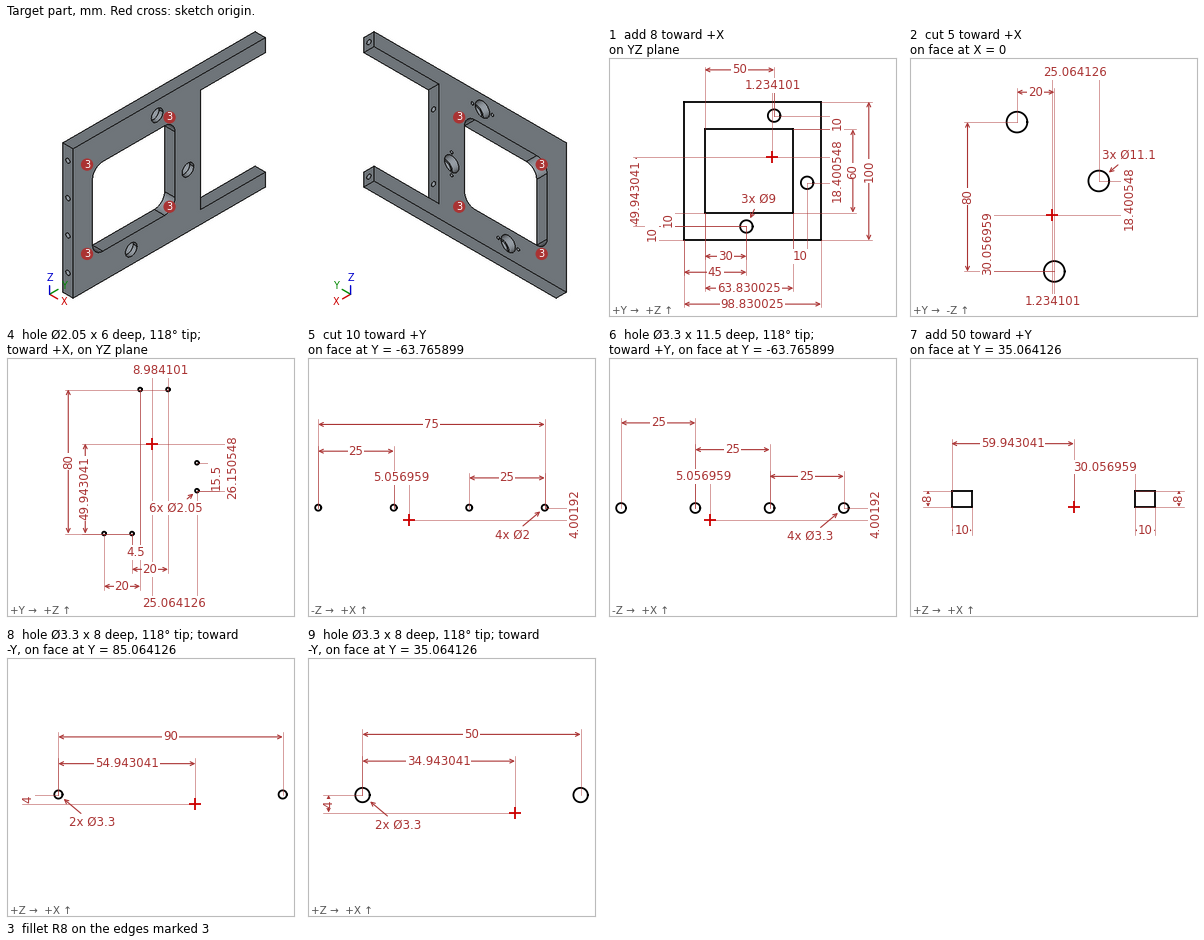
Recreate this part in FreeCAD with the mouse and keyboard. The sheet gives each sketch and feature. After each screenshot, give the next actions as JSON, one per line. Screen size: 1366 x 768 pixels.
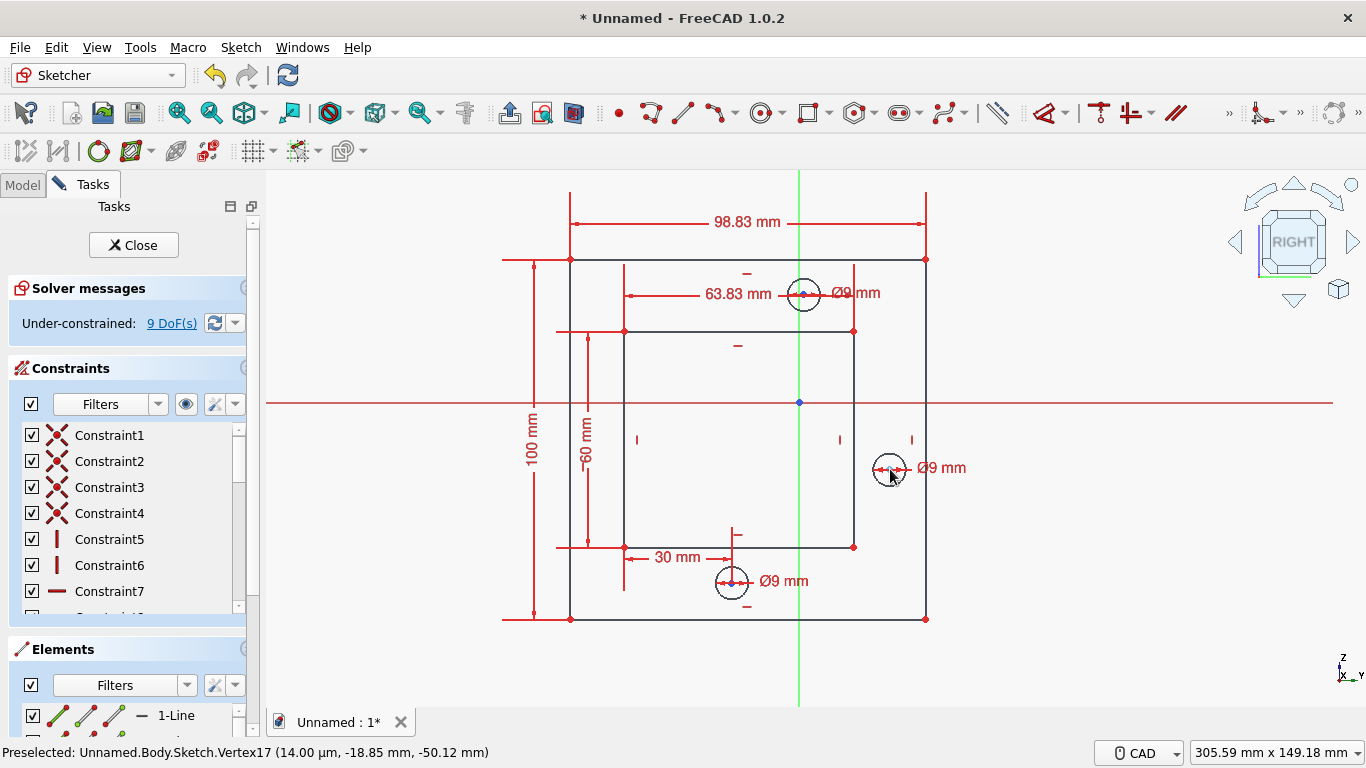
{"action": "left_click", "coordinate": [570, 620]}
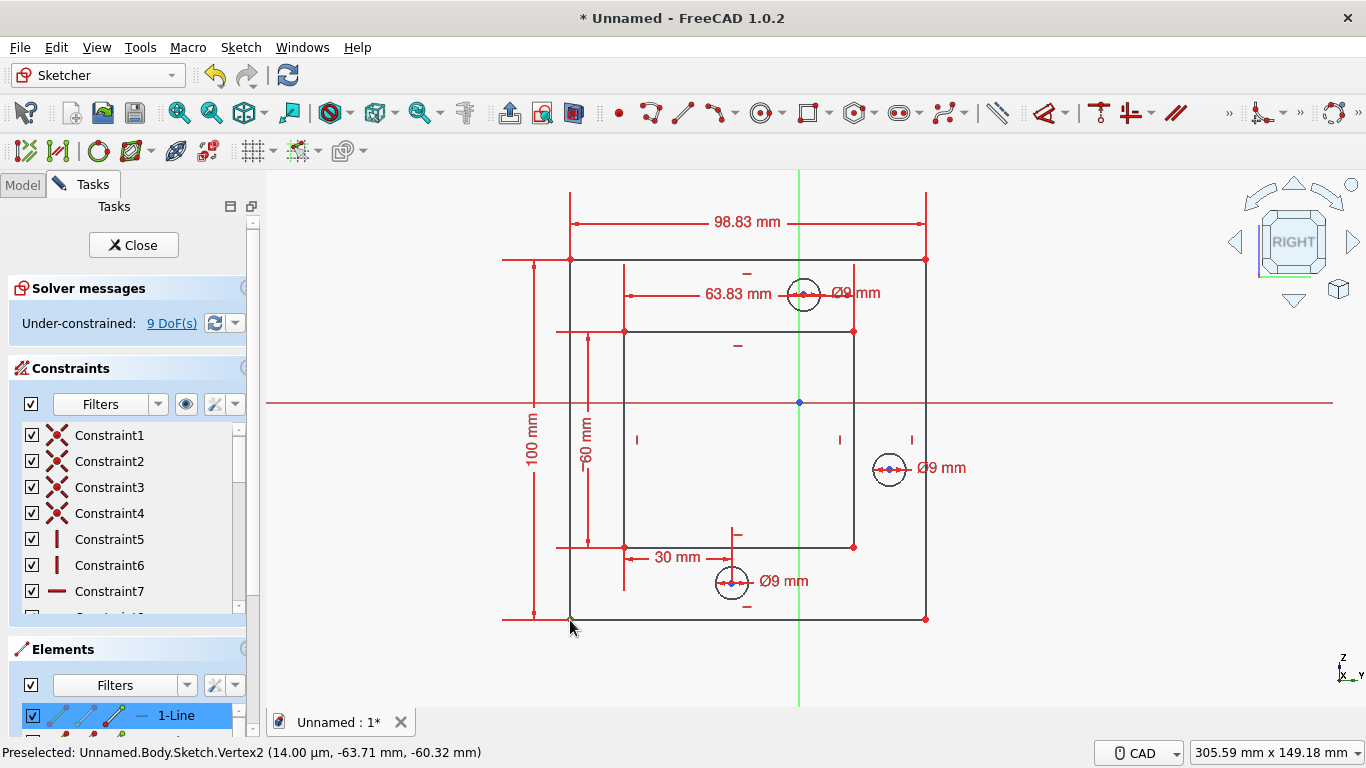
{"action": "left_click", "coordinate": [732, 583]}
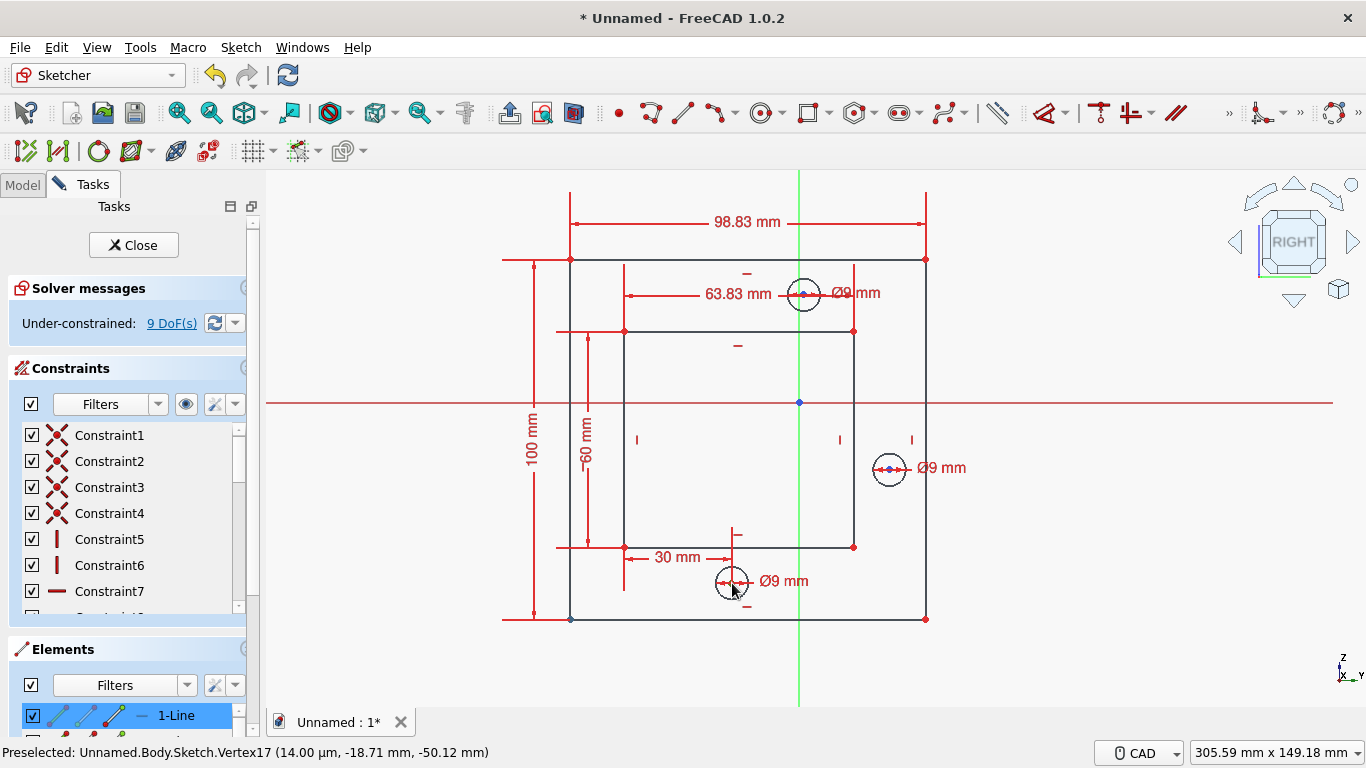
{"action": "key", "text": "l"}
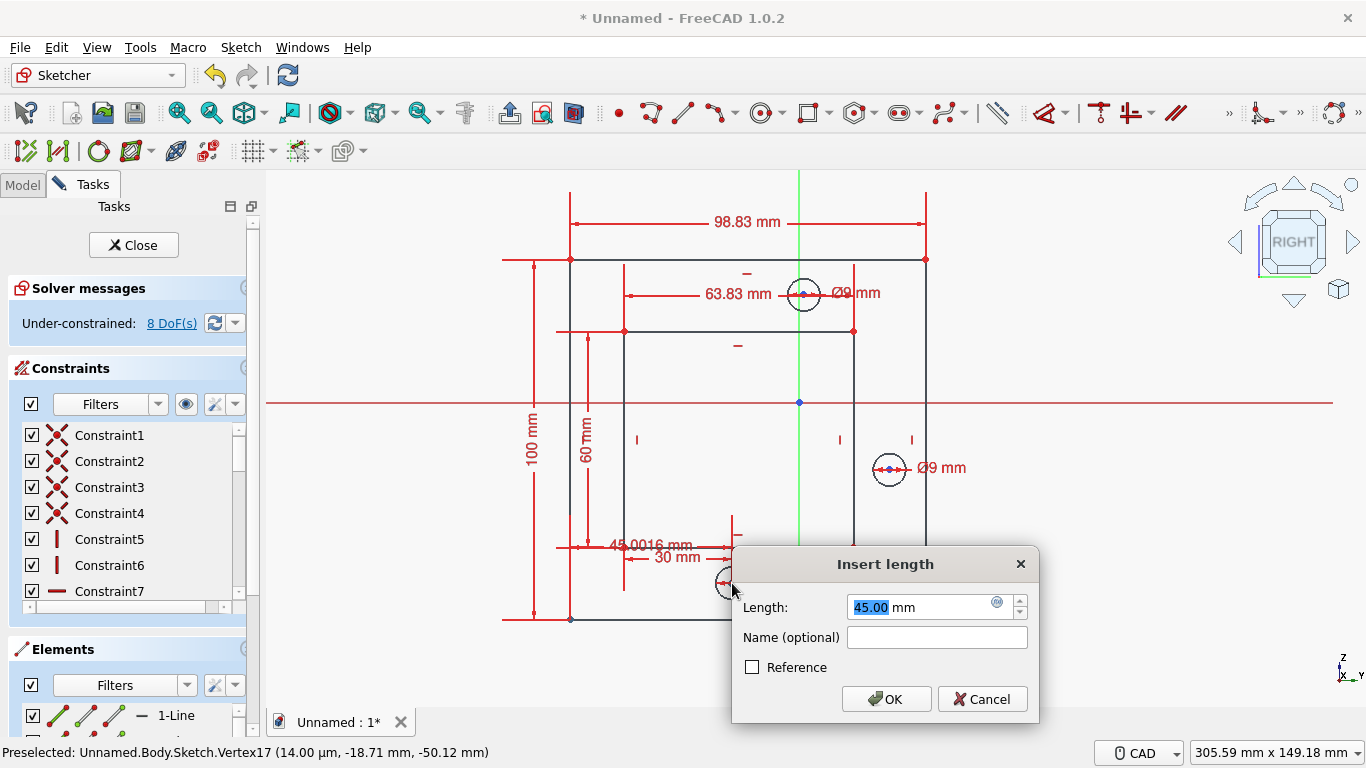
{"action": "type", "text": "45"}
{"action": "key", "text": "Return"}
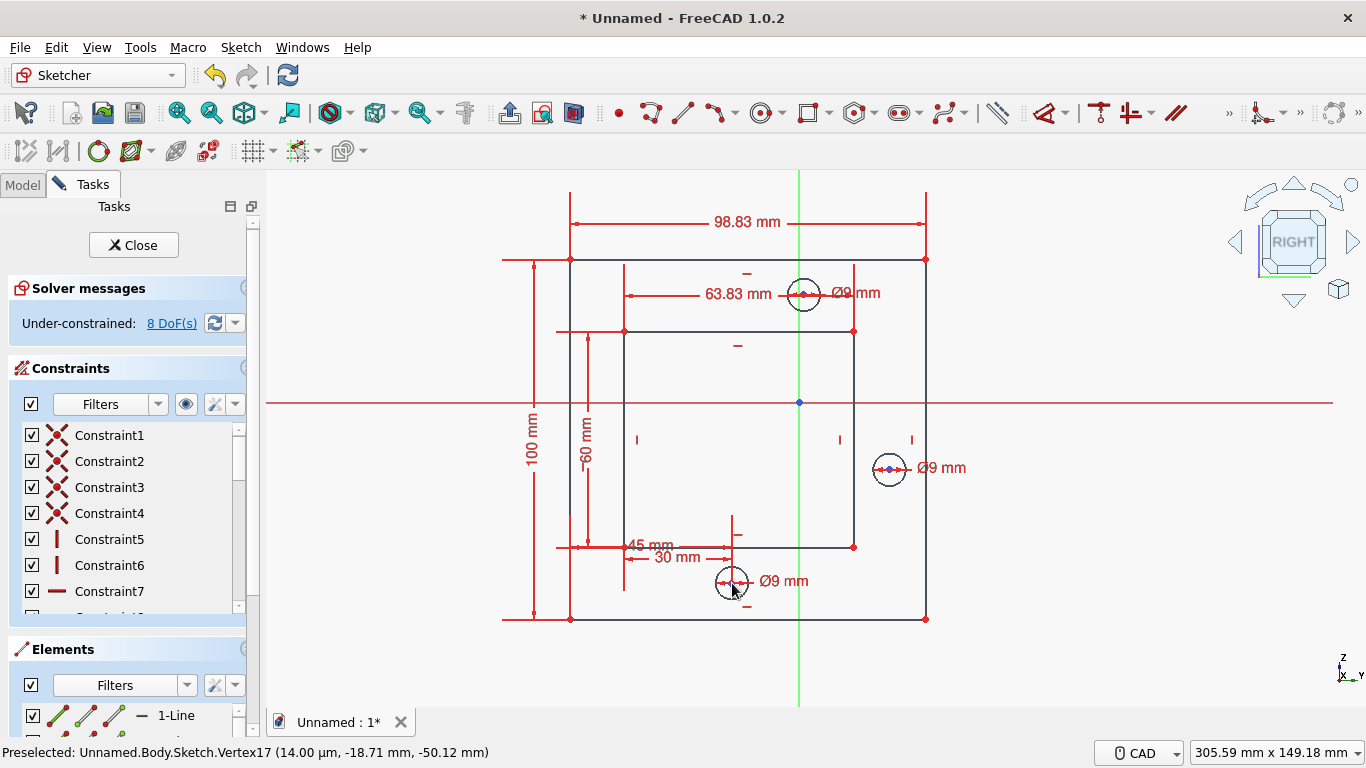
{"action": "left_click", "coordinate": [624, 548]}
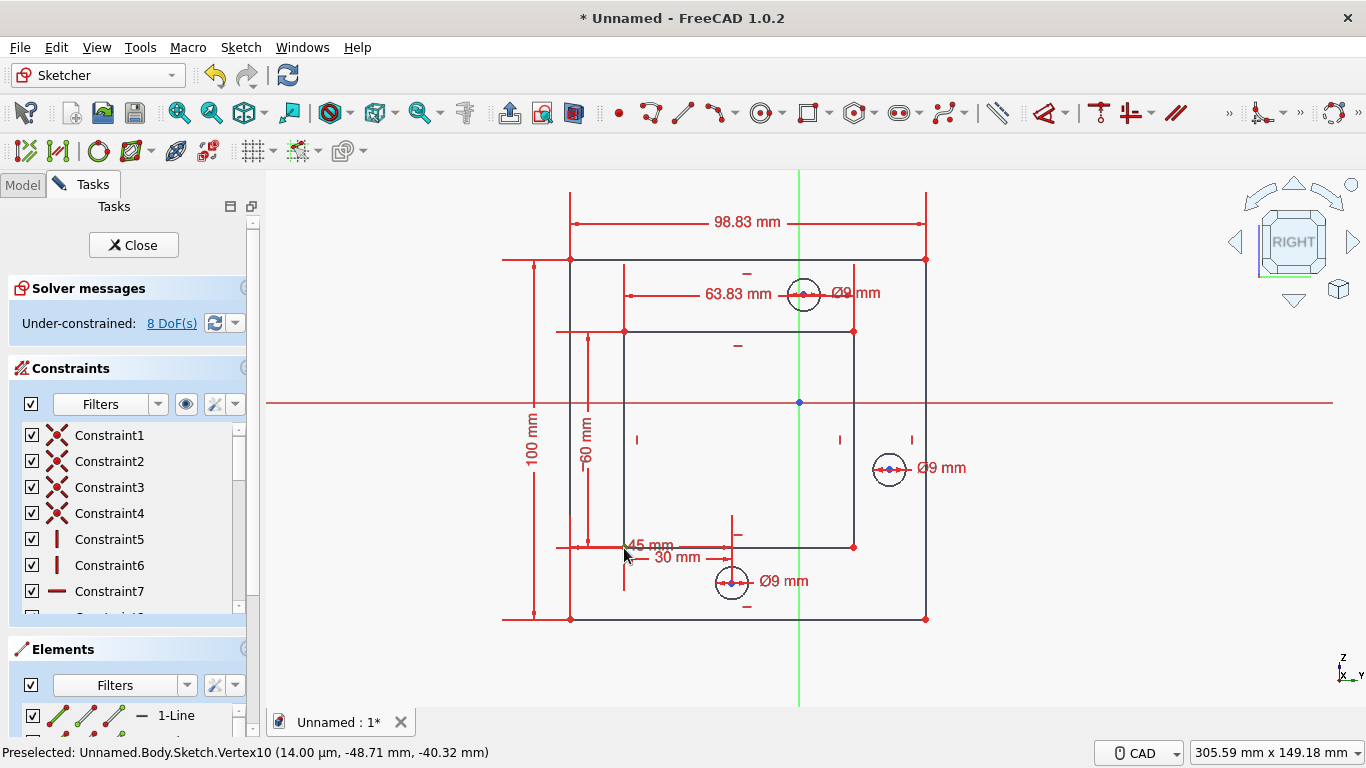
{"action": "left_click", "coordinate": [732, 583]}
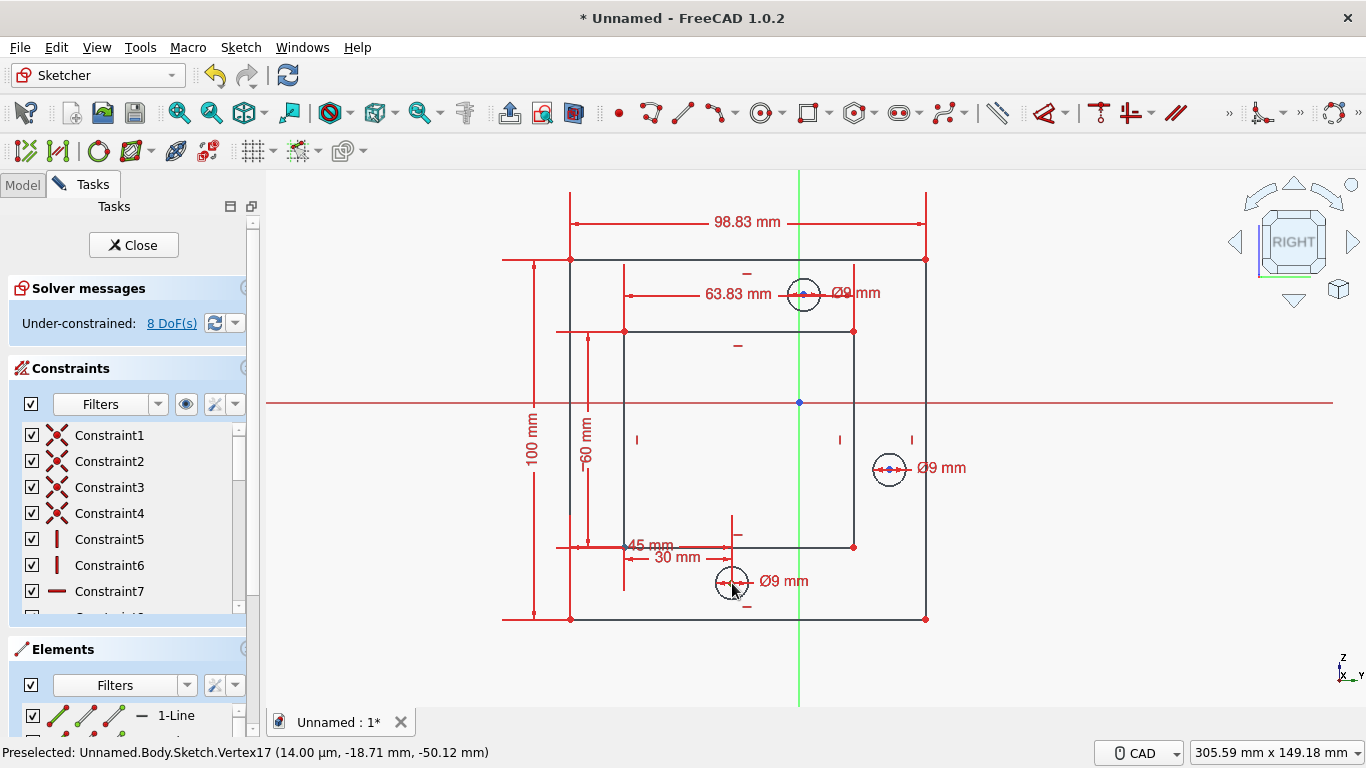
{"action": "key", "text": "i"}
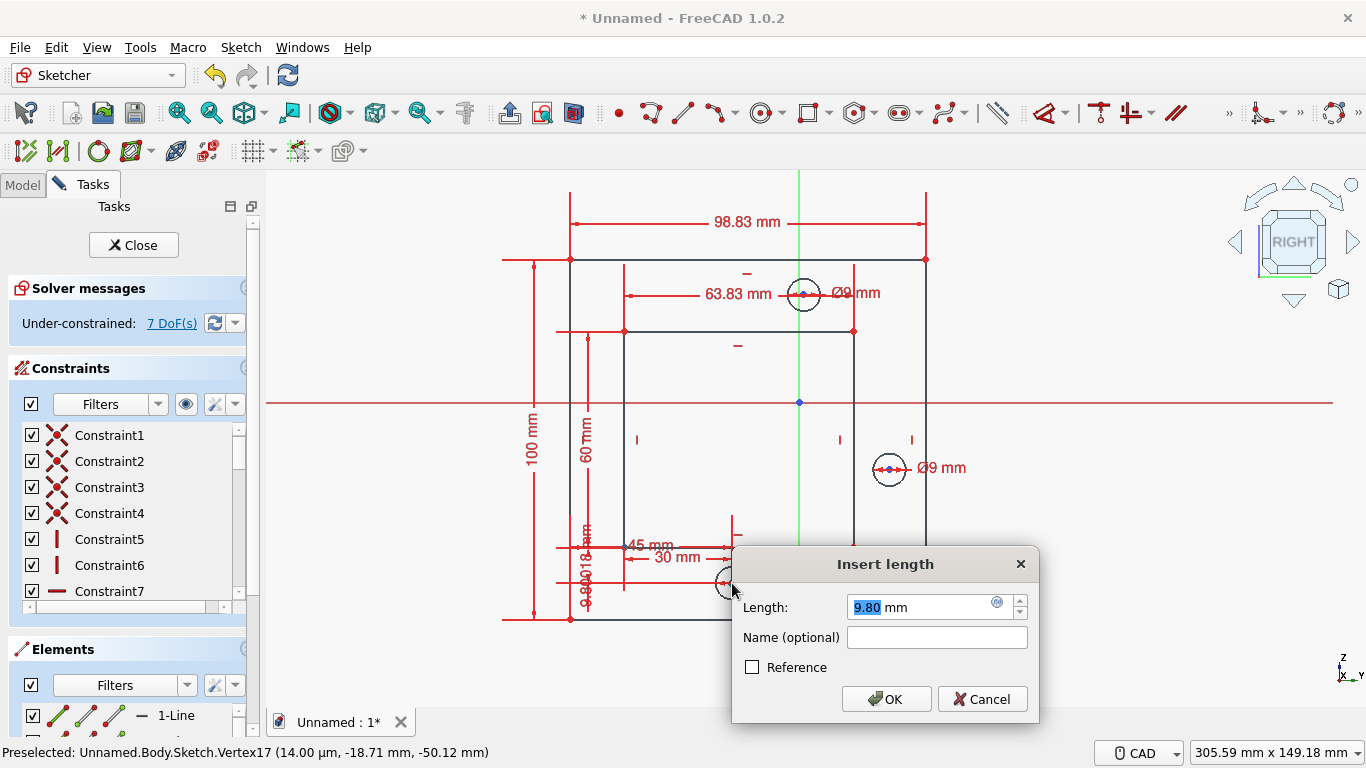
{"action": "type", "text": "10"}
{"action": "key", "text": "Return"}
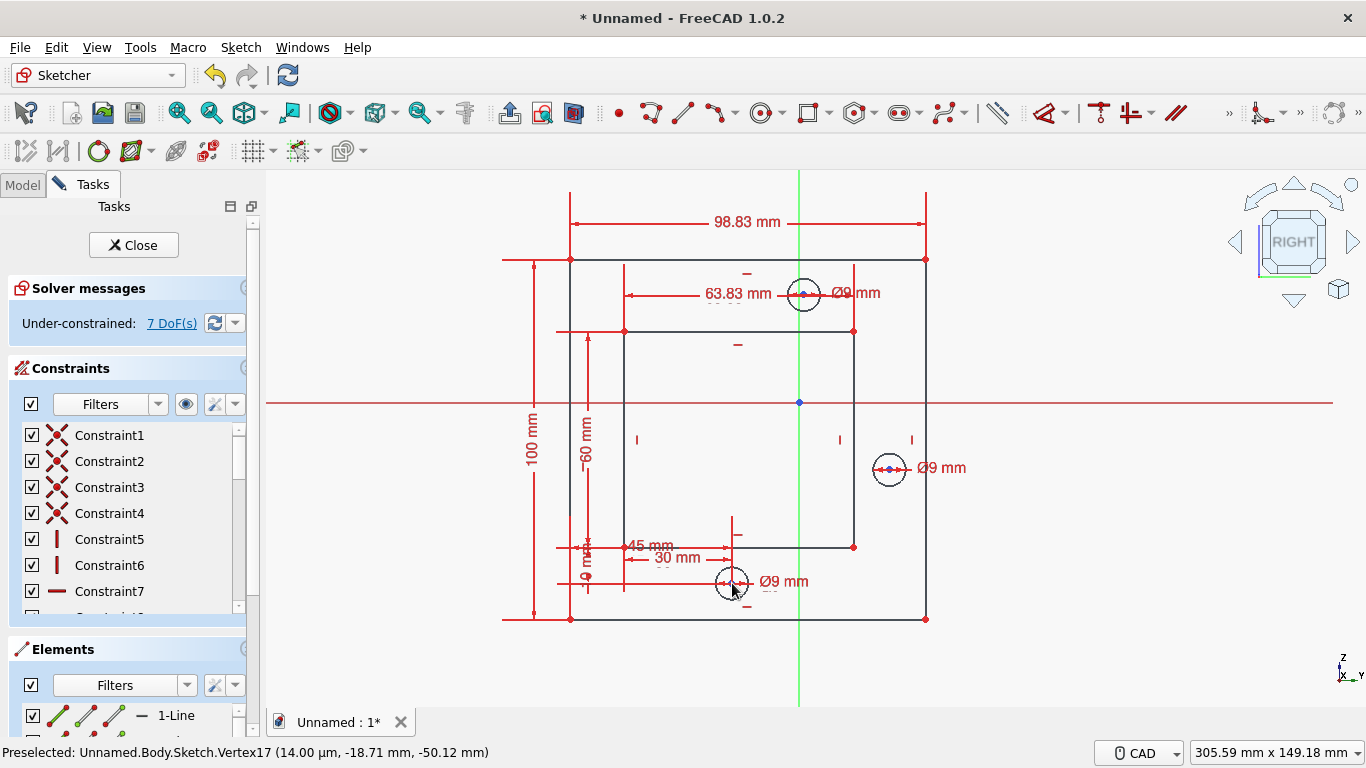
{"action": "left_click", "coordinate": [570, 620]}